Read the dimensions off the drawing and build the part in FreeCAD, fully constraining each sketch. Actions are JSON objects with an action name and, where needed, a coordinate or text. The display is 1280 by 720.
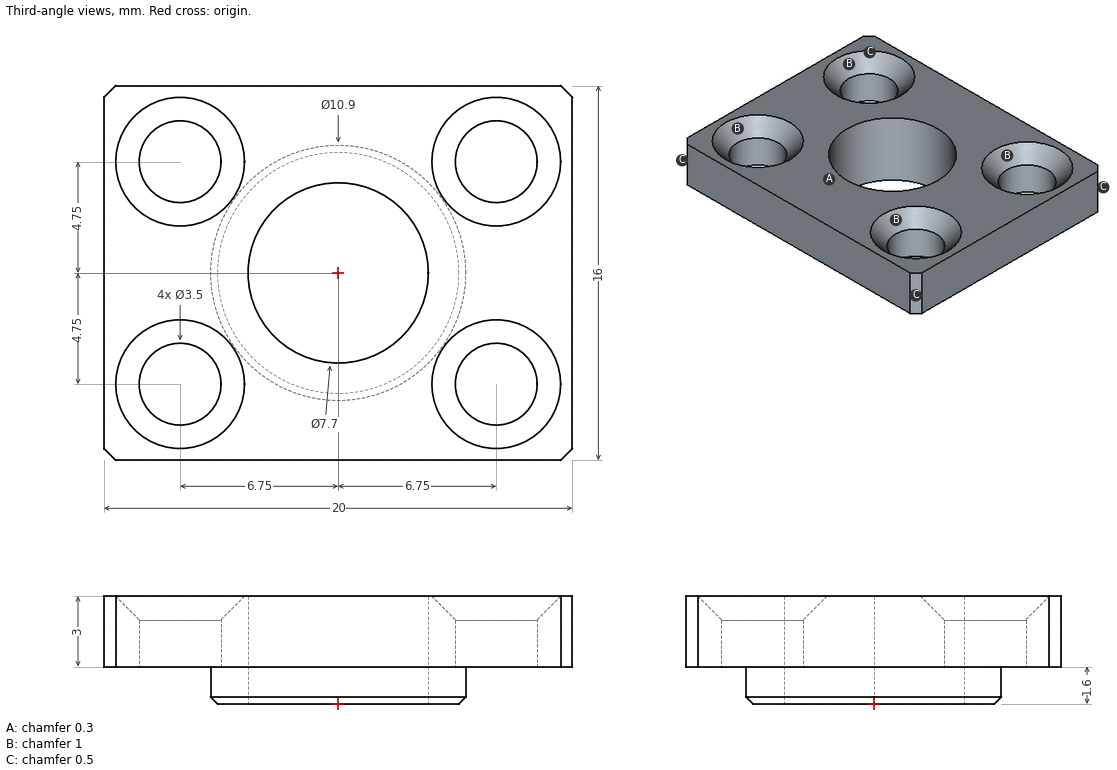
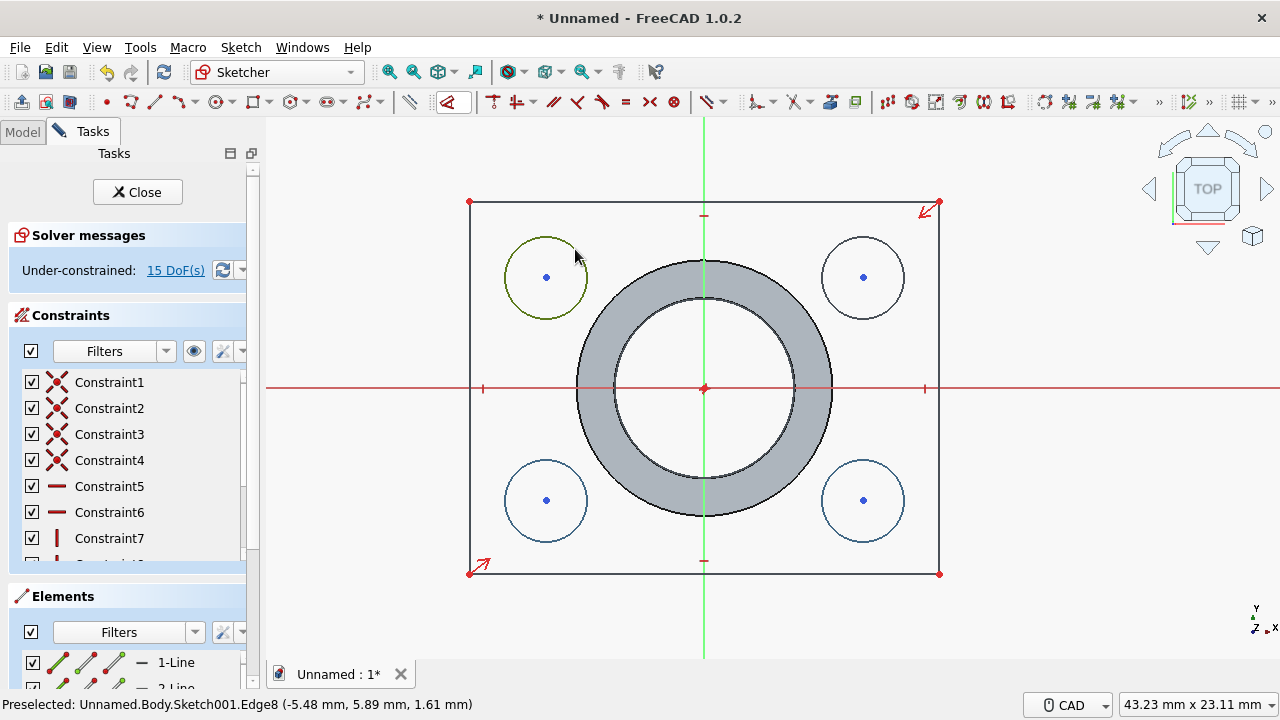
{"action": "left_click", "coordinate": [892, 249]}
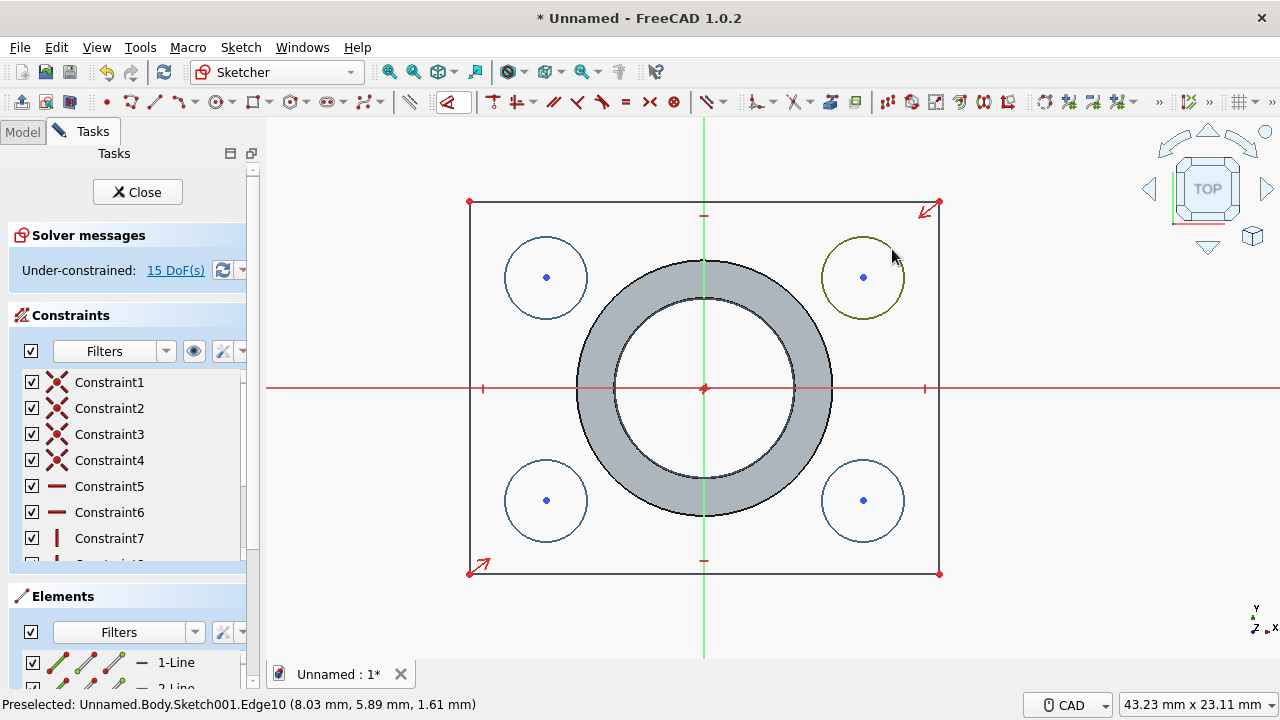
{"action": "key", "text": "e"}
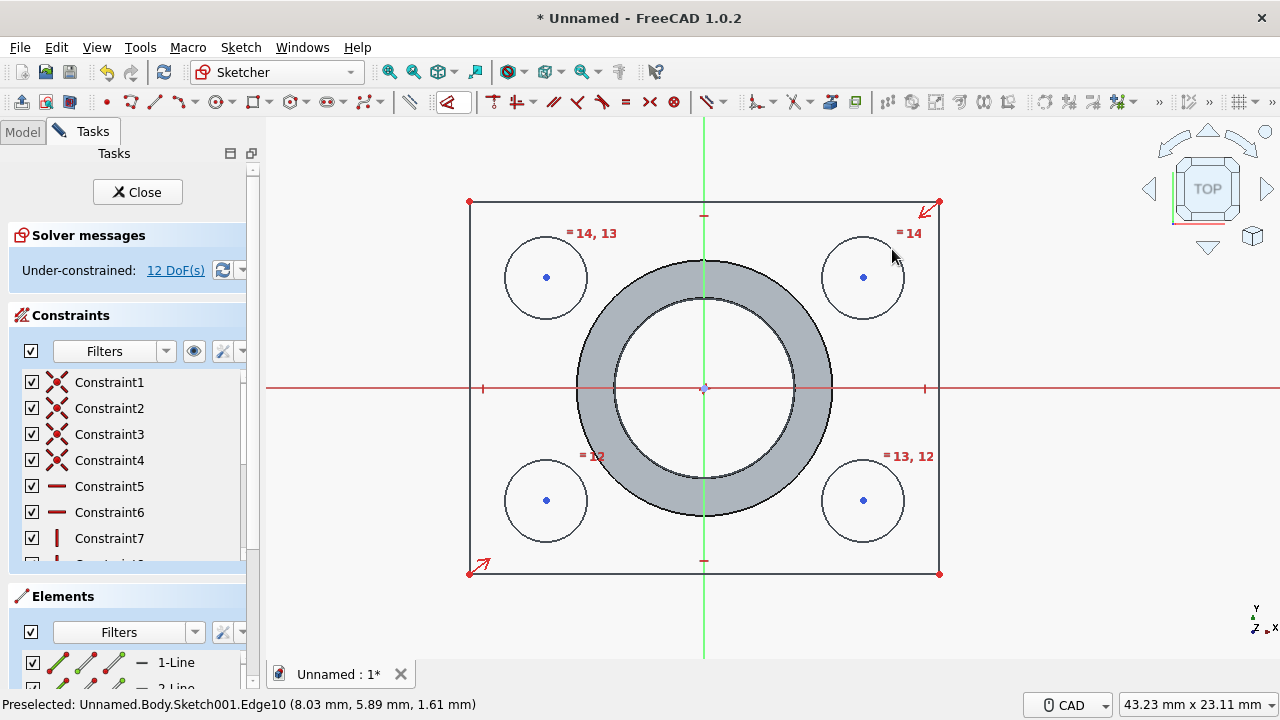
{"action": "left_click", "coordinate": [546, 501]}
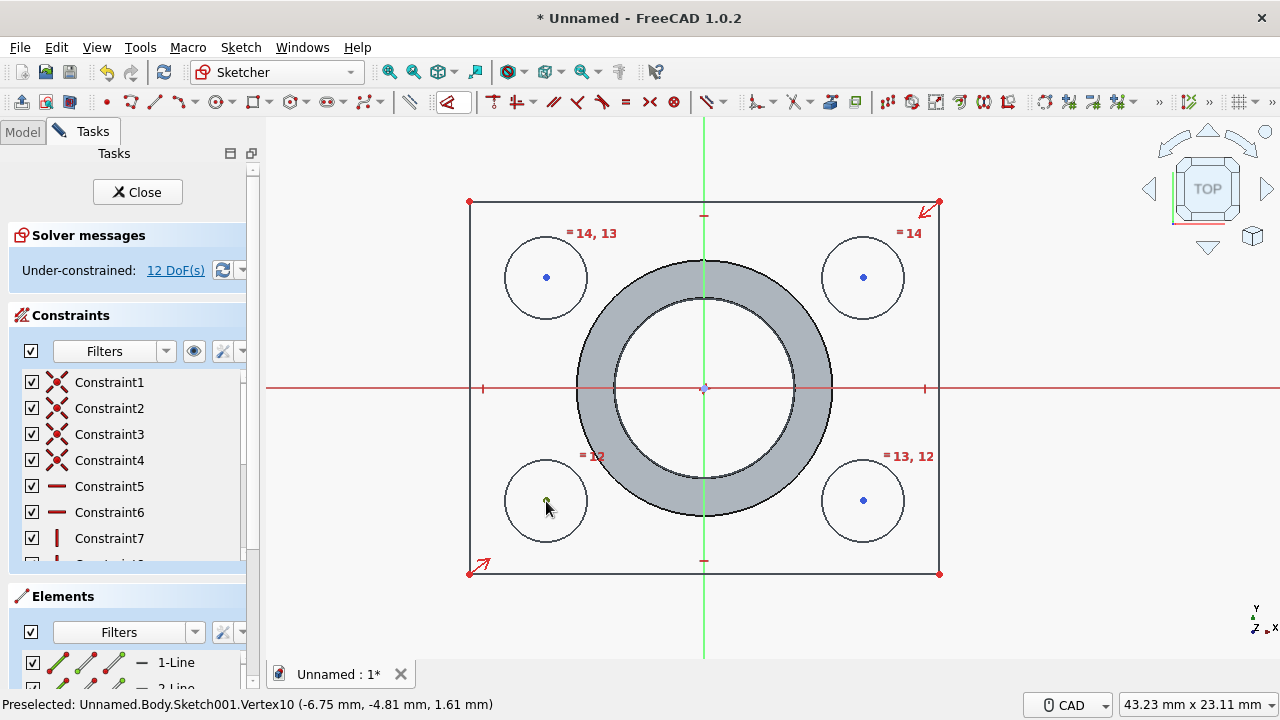
{"action": "left_click", "coordinate": [863, 501]}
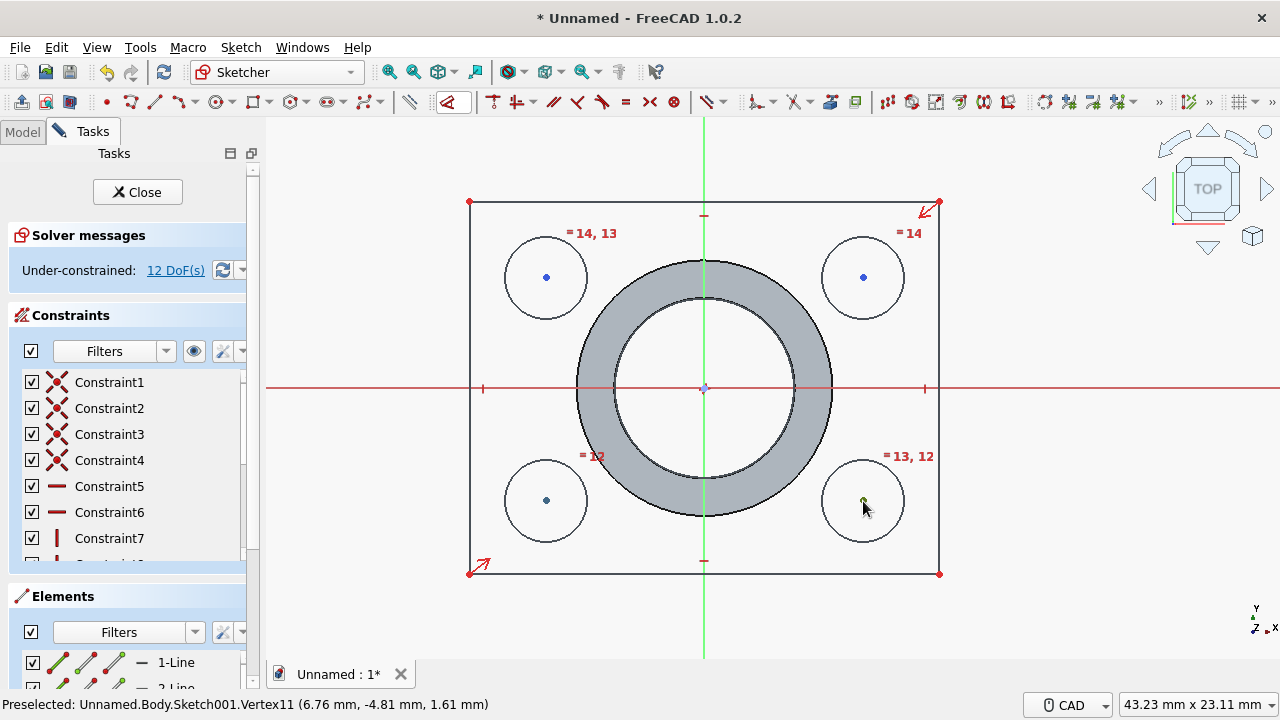
{"action": "key", "text": "h"}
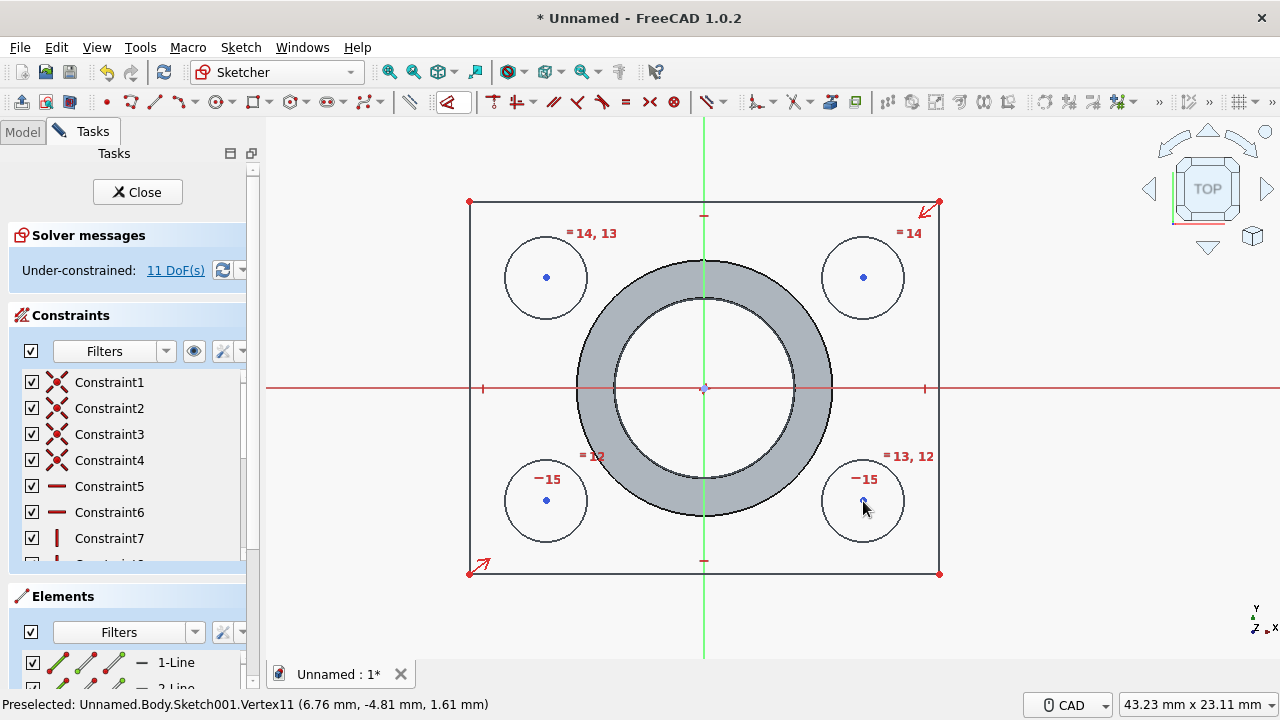
{"action": "left_click", "coordinate": [546, 501]}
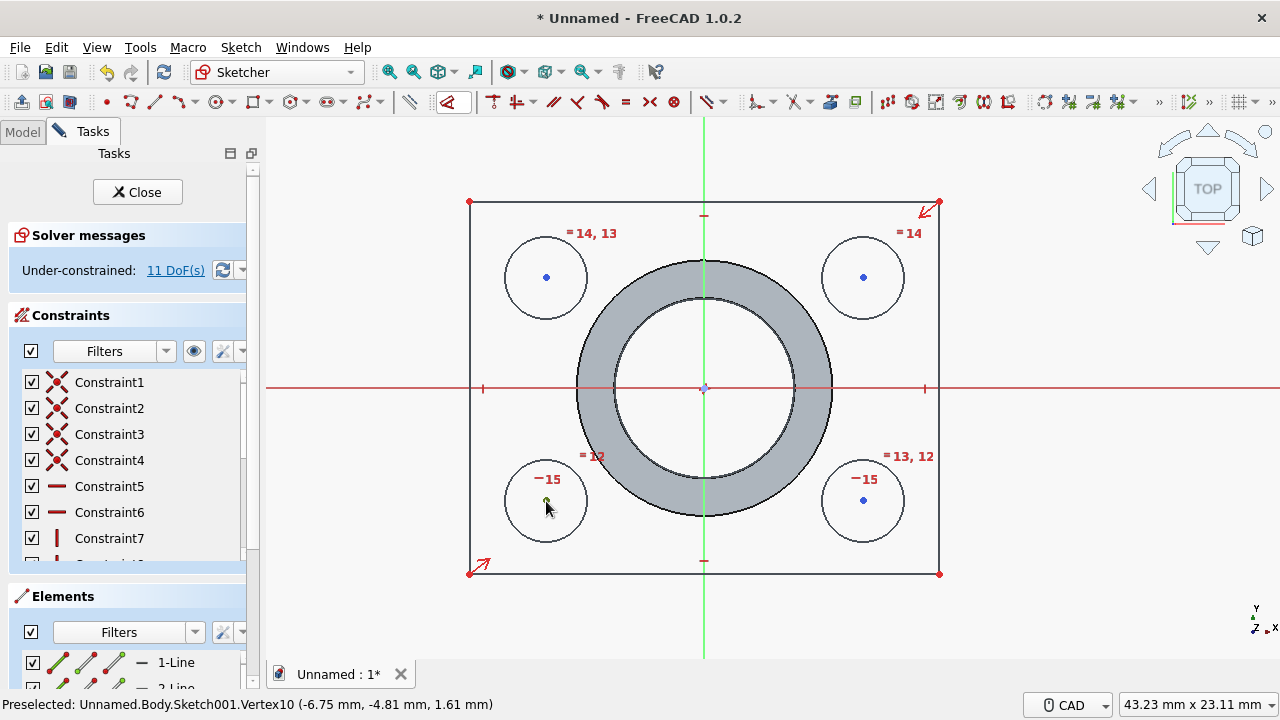
{"action": "left_click", "coordinate": [546, 278]}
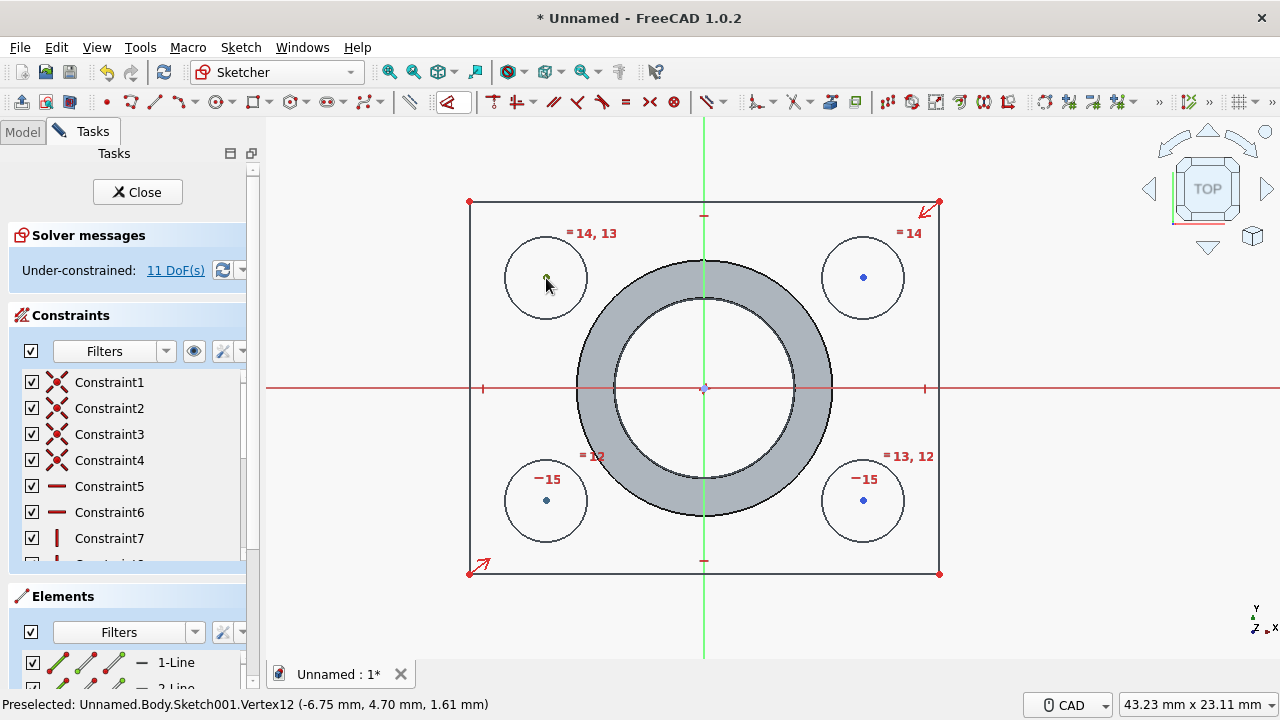
{"action": "key", "text": "v"}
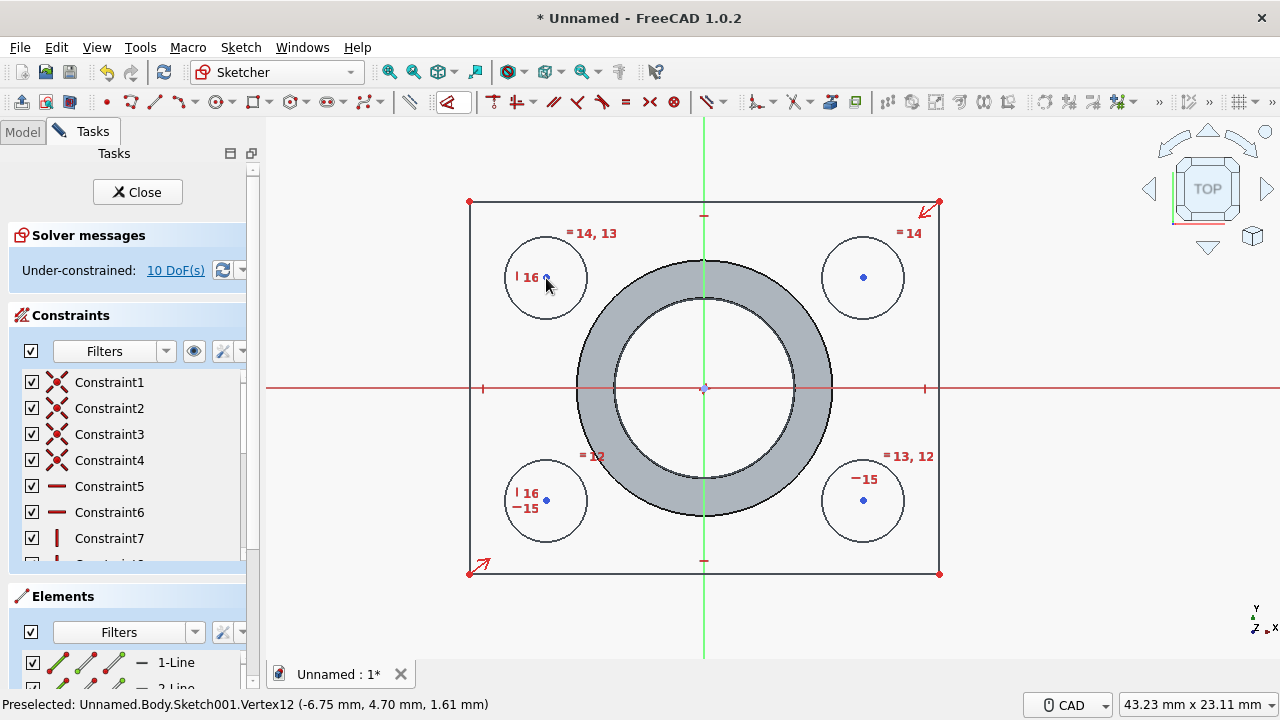
{"action": "left_click", "coordinate": [863, 501]}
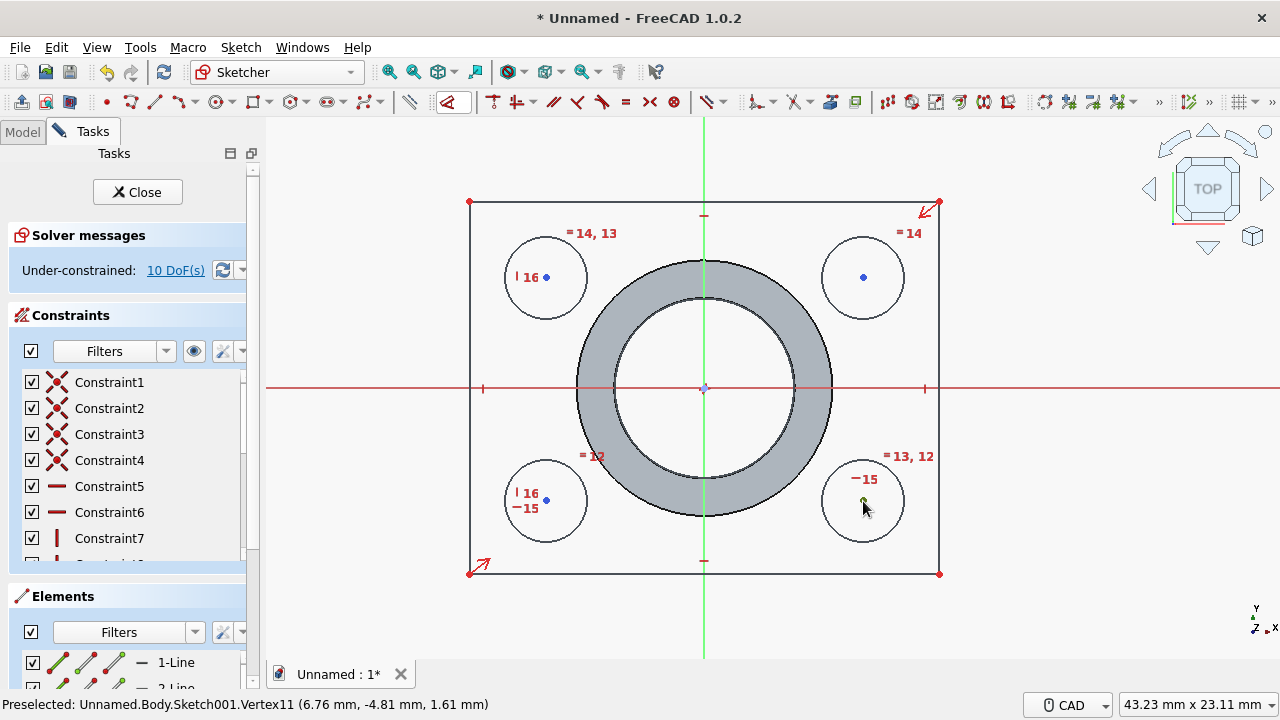
{"action": "left_click", "coordinate": [863, 278]}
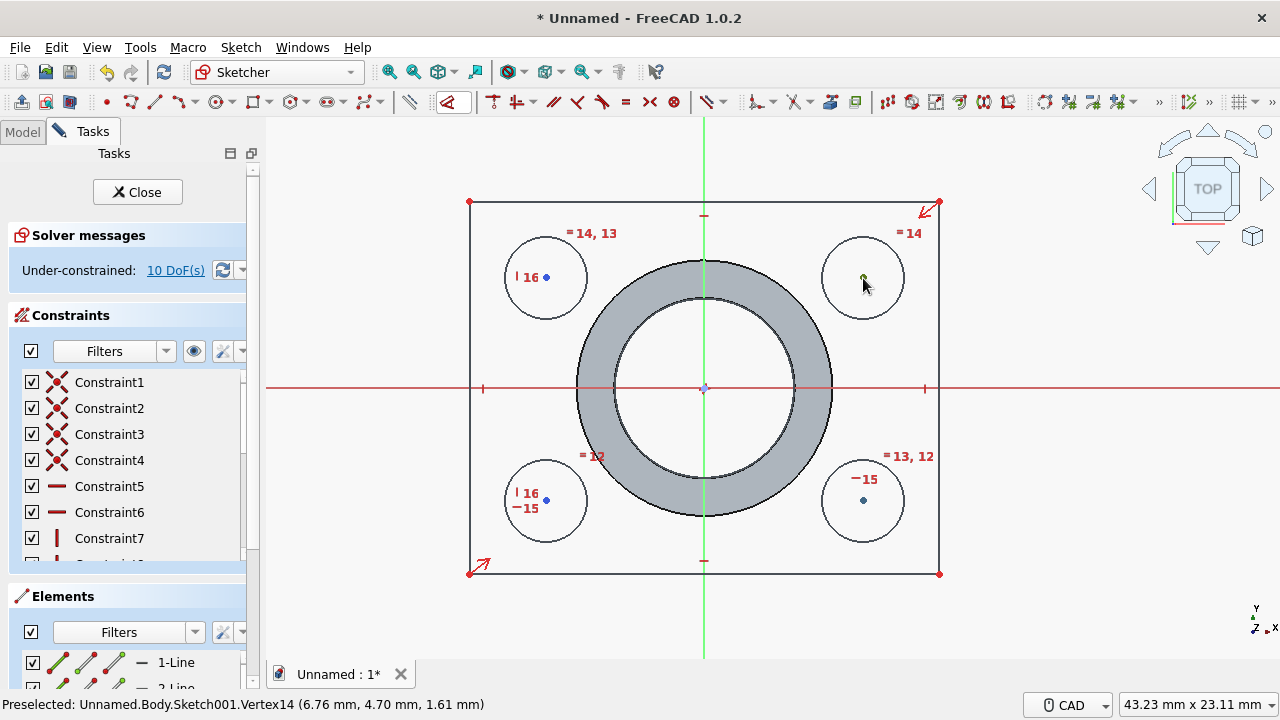
{"action": "key", "text": "v"}